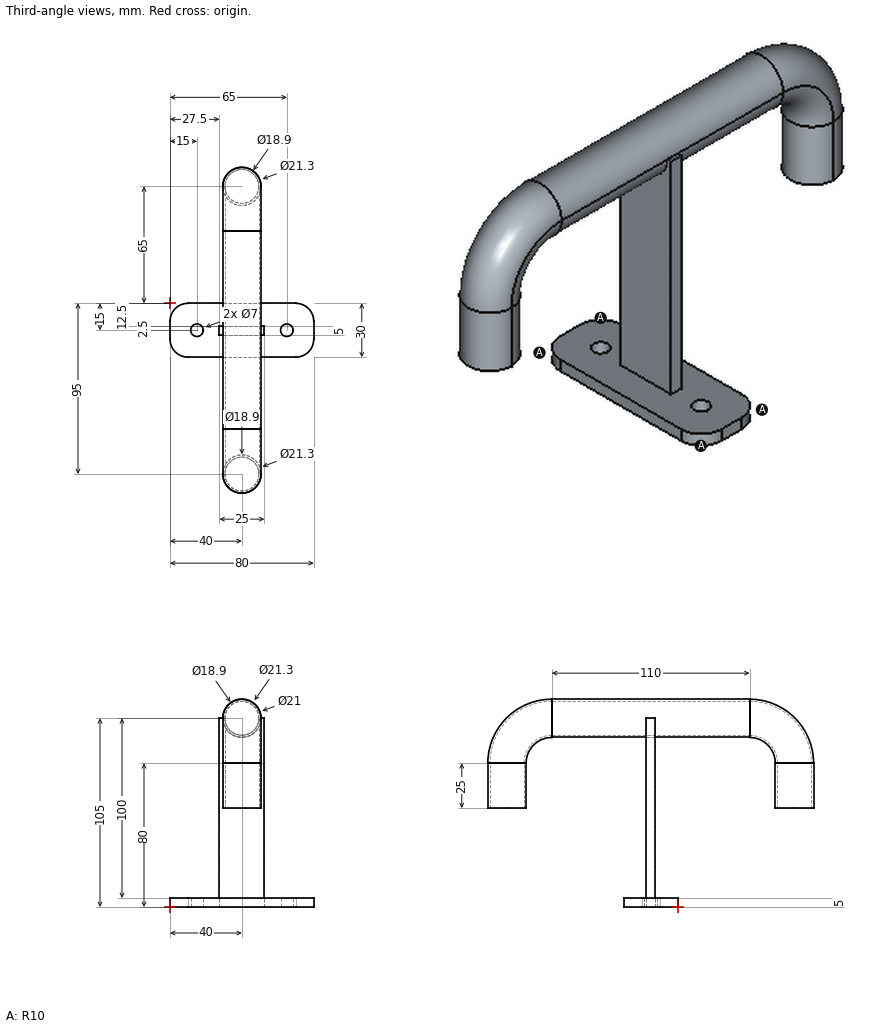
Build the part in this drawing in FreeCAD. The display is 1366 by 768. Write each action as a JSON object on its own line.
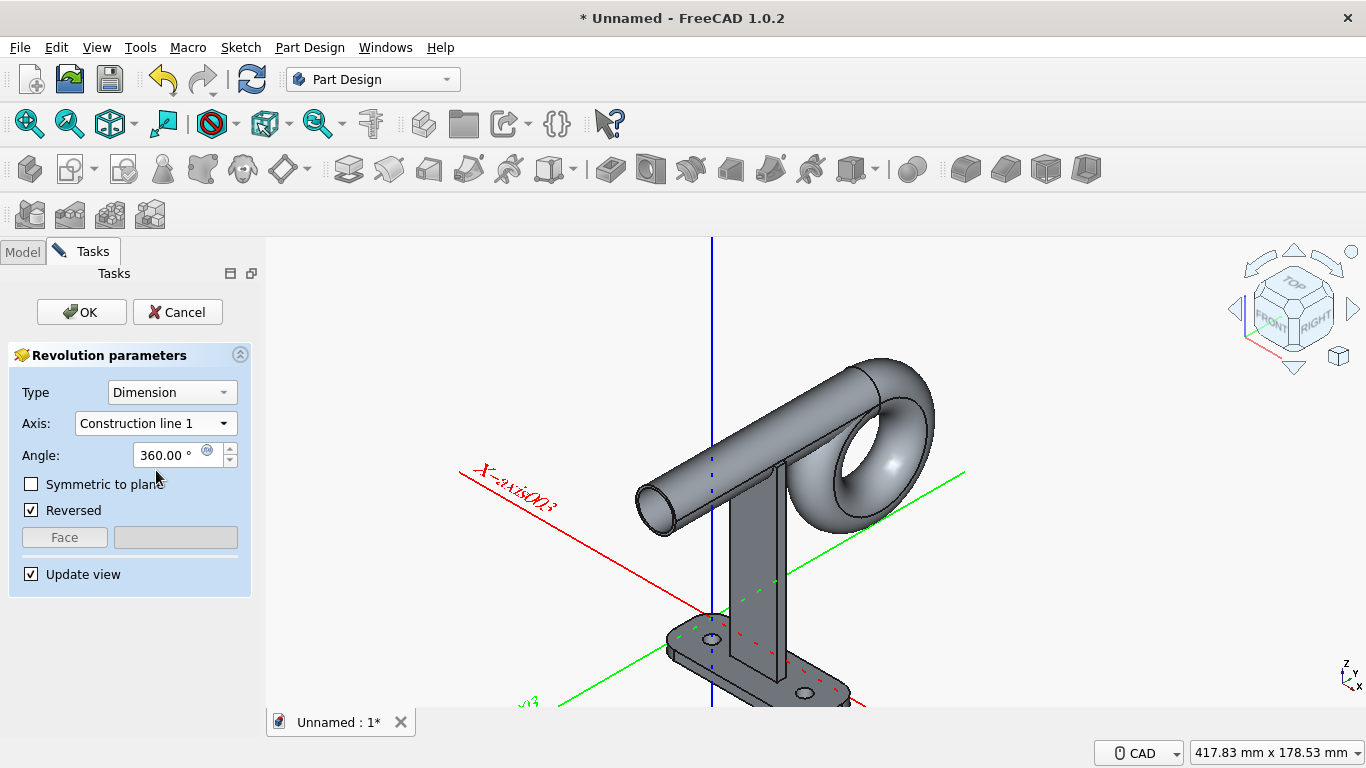
{"action": "triple_click", "coordinate": [178, 455]}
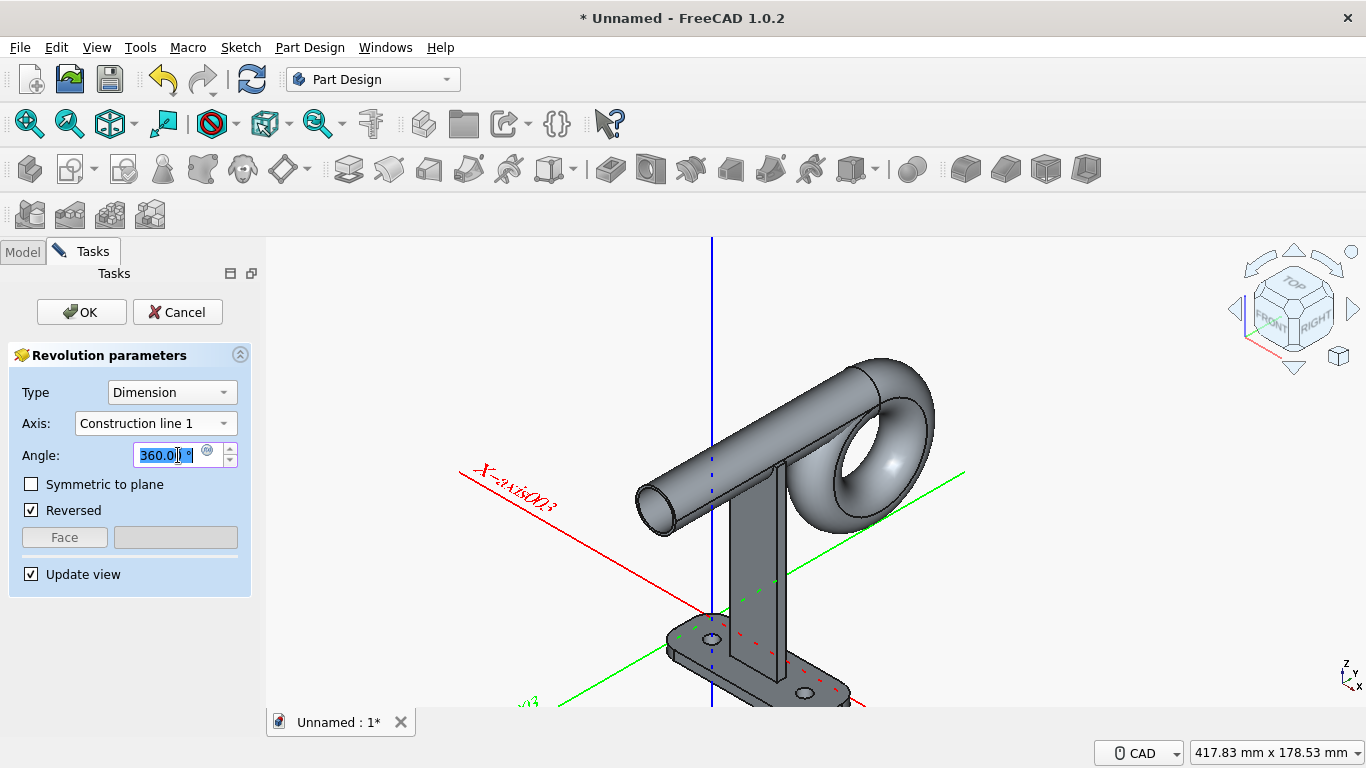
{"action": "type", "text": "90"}
{"action": "key", "text": "Tab"}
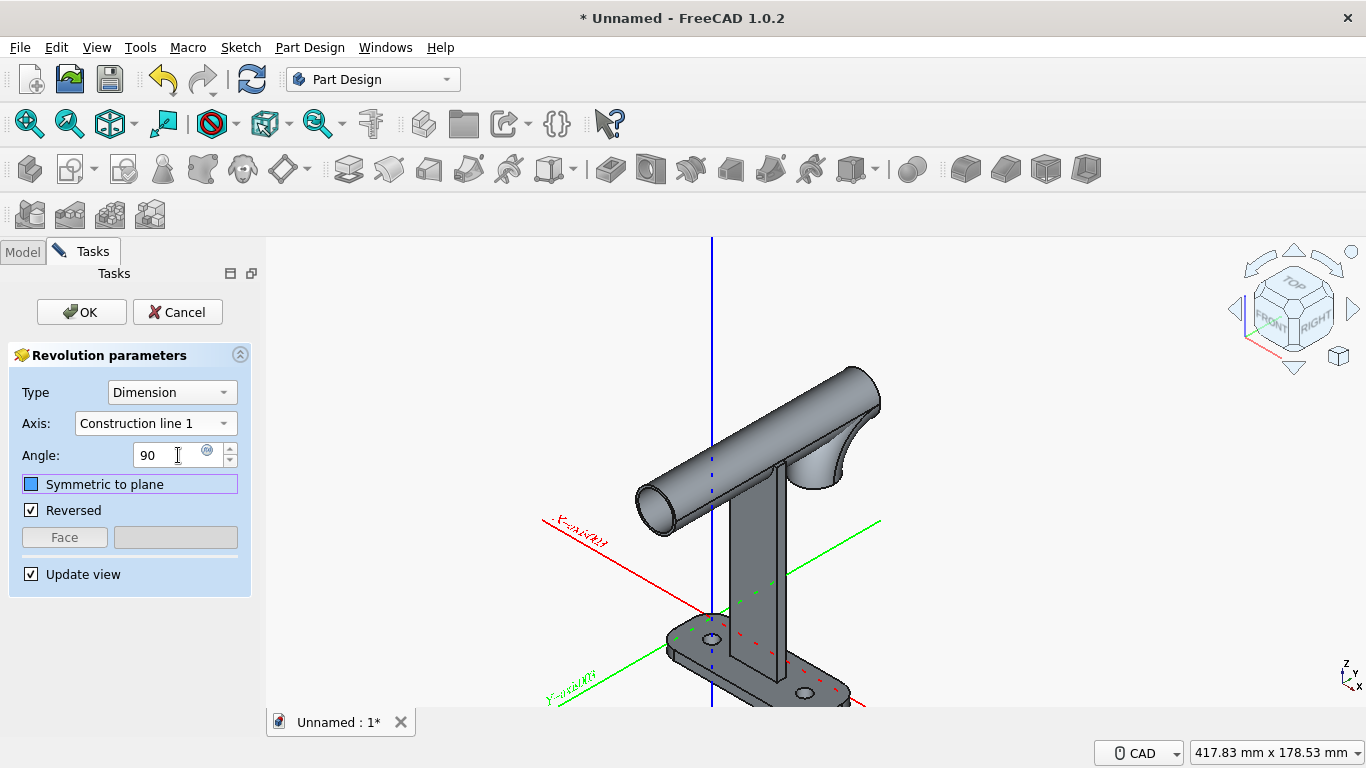
{"action": "left_click", "coordinate": [30, 510]}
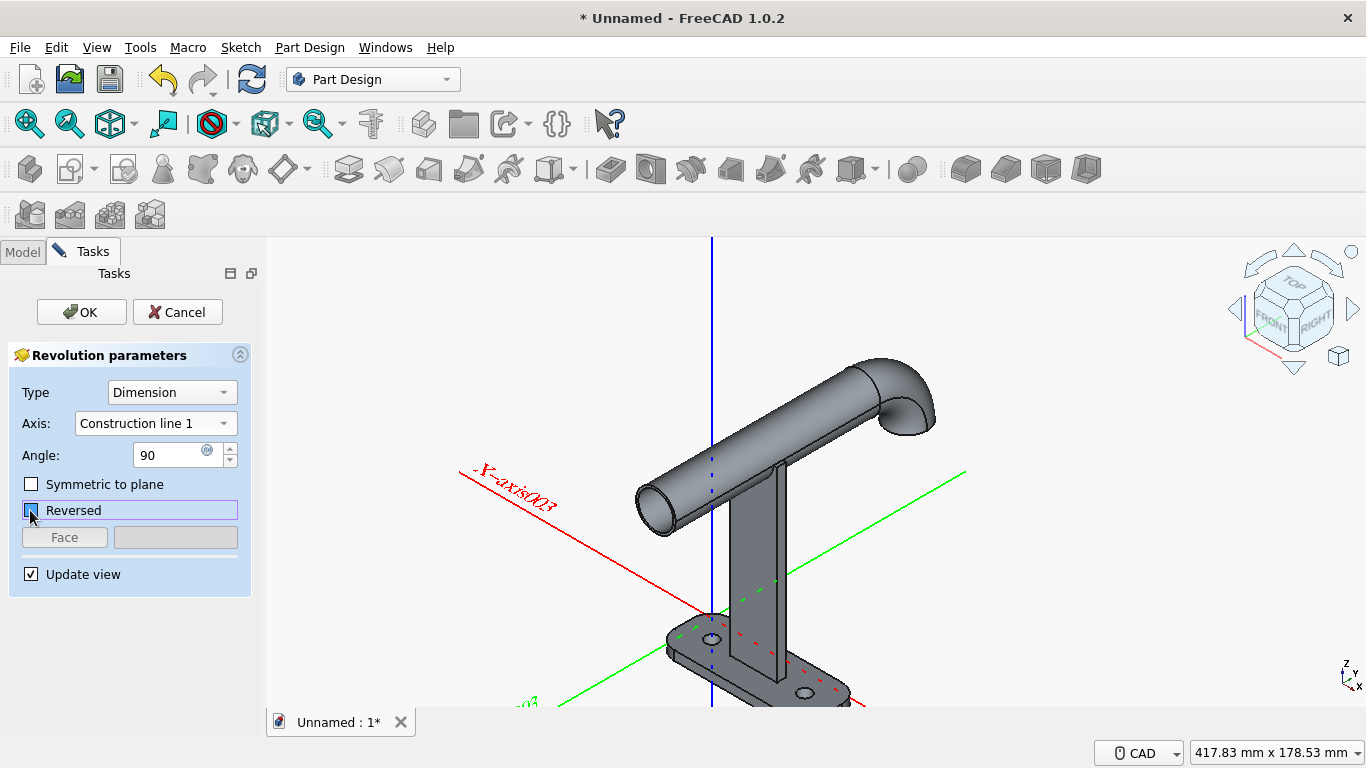
{"action": "left_click", "coordinate": [82, 312]}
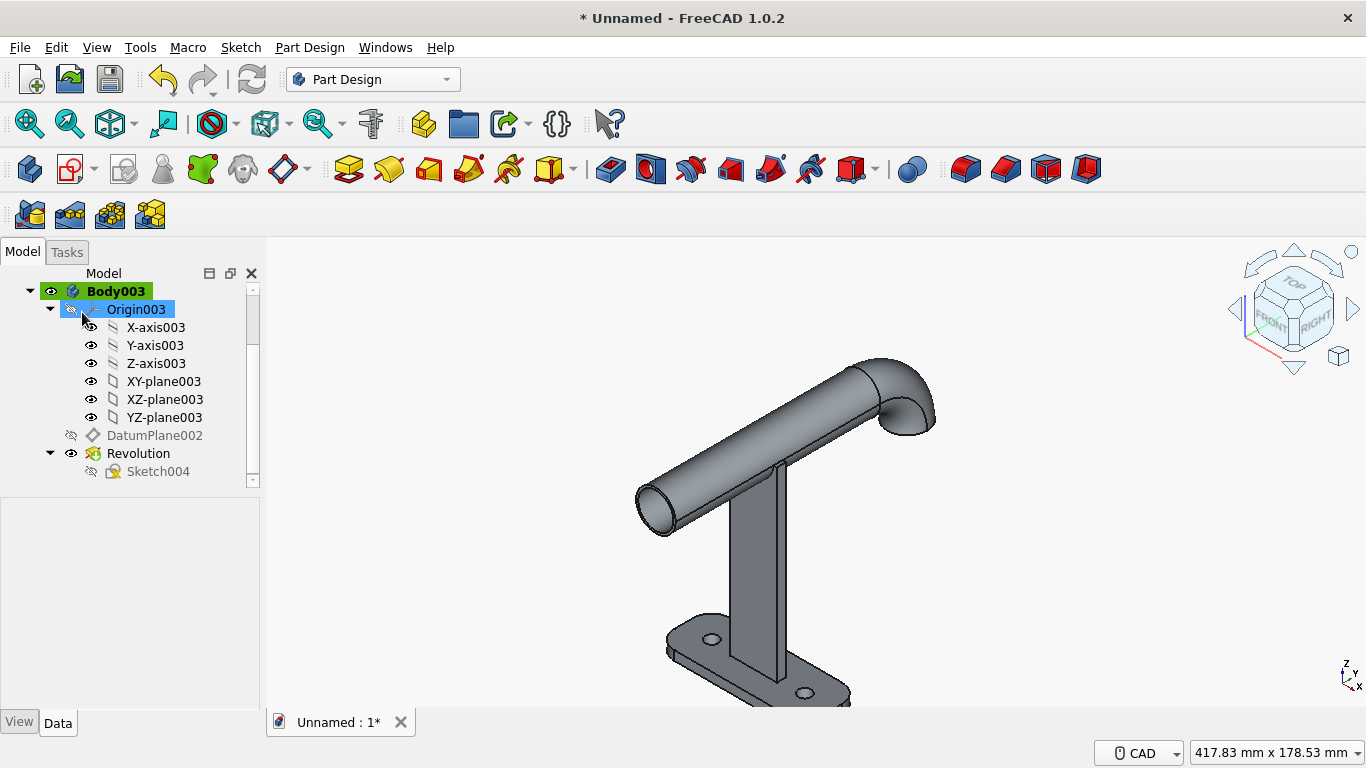
{"action": "left_click", "coordinate": [30, 124]}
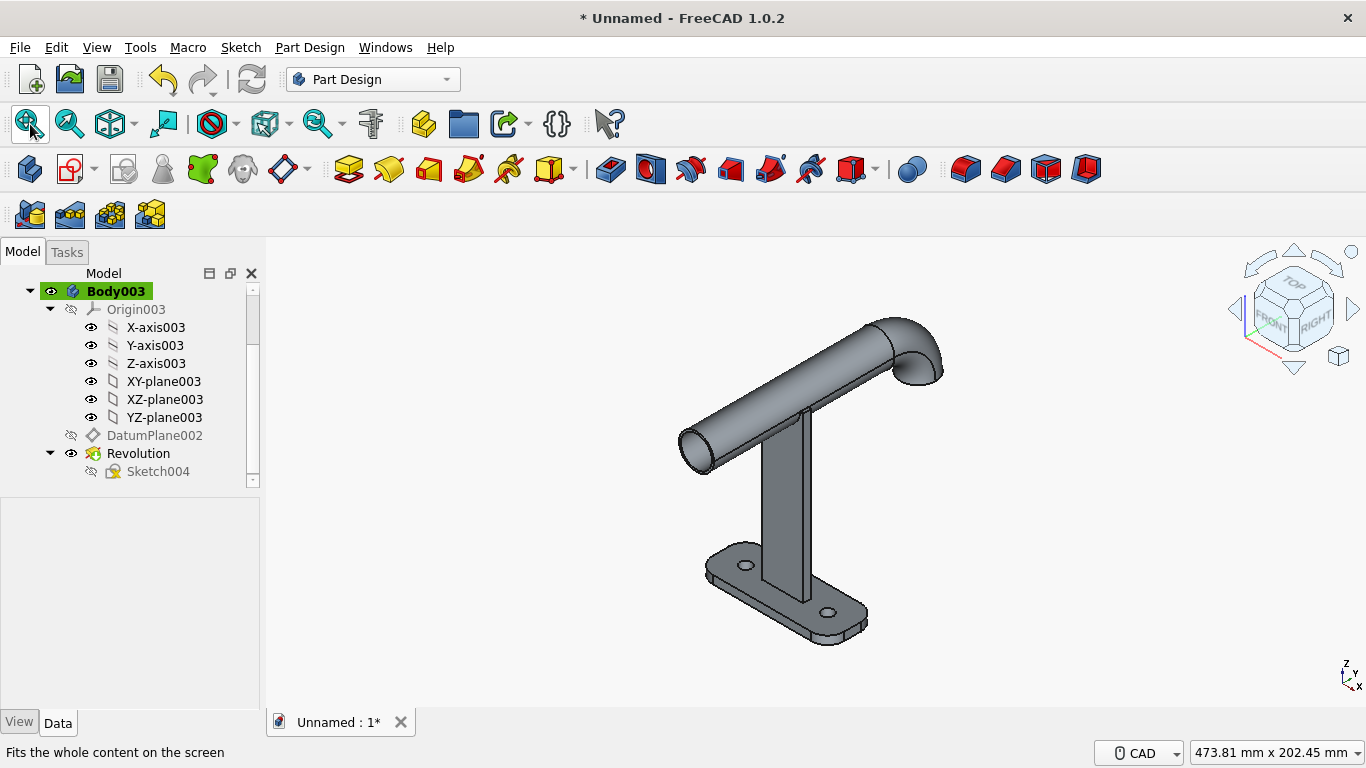
{"action": "left_click", "coordinate": [30, 170]}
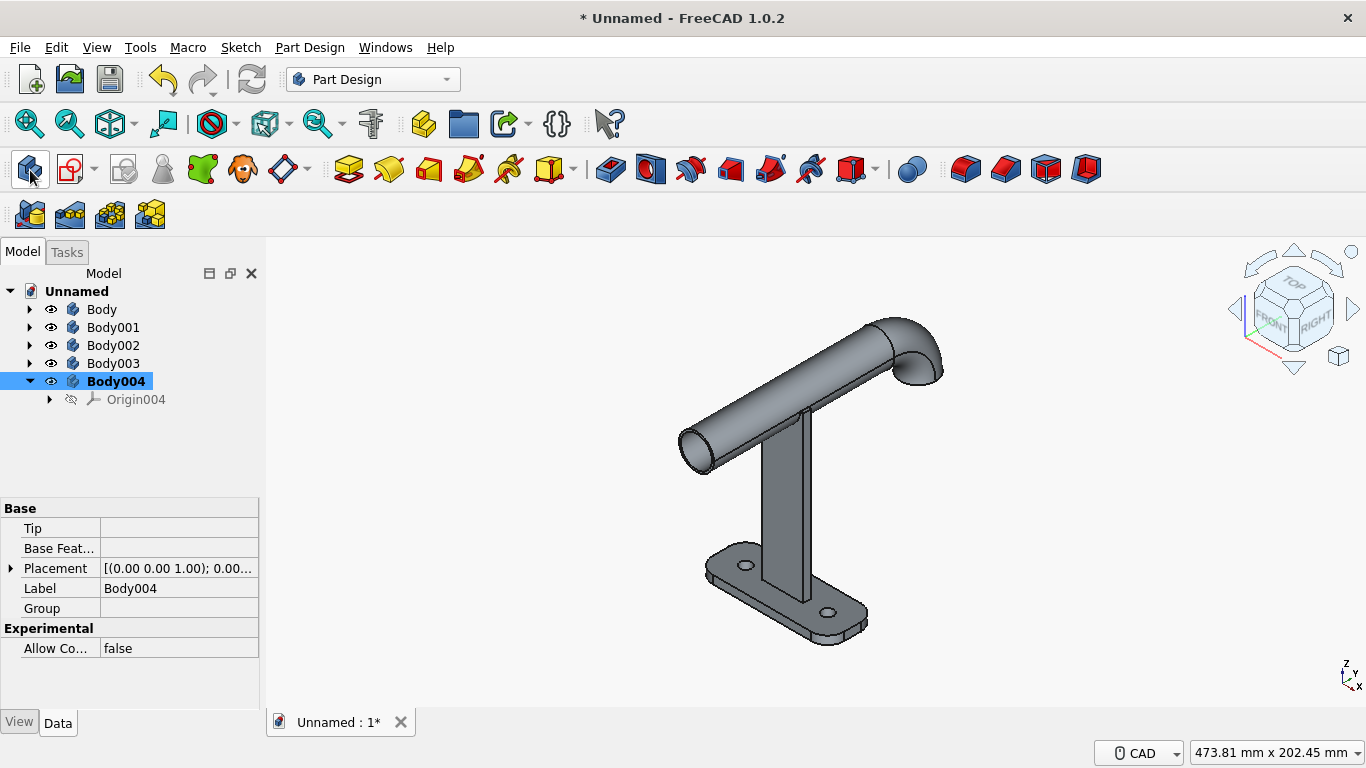
{"action": "left_click", "coordinate": [50, 399]}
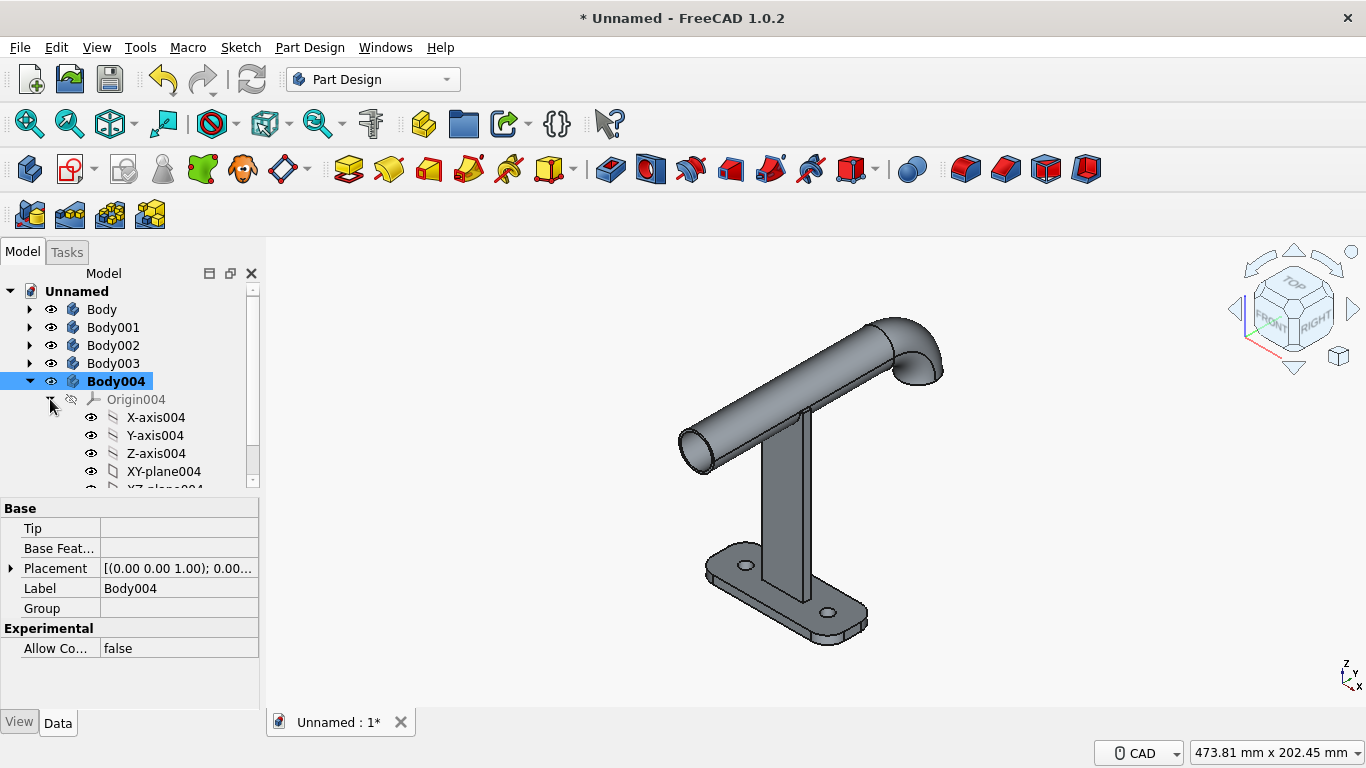
{"action": "scroll", "coordinate": [100, 377], "scroll_direction": "down", "scroll_amount": 3}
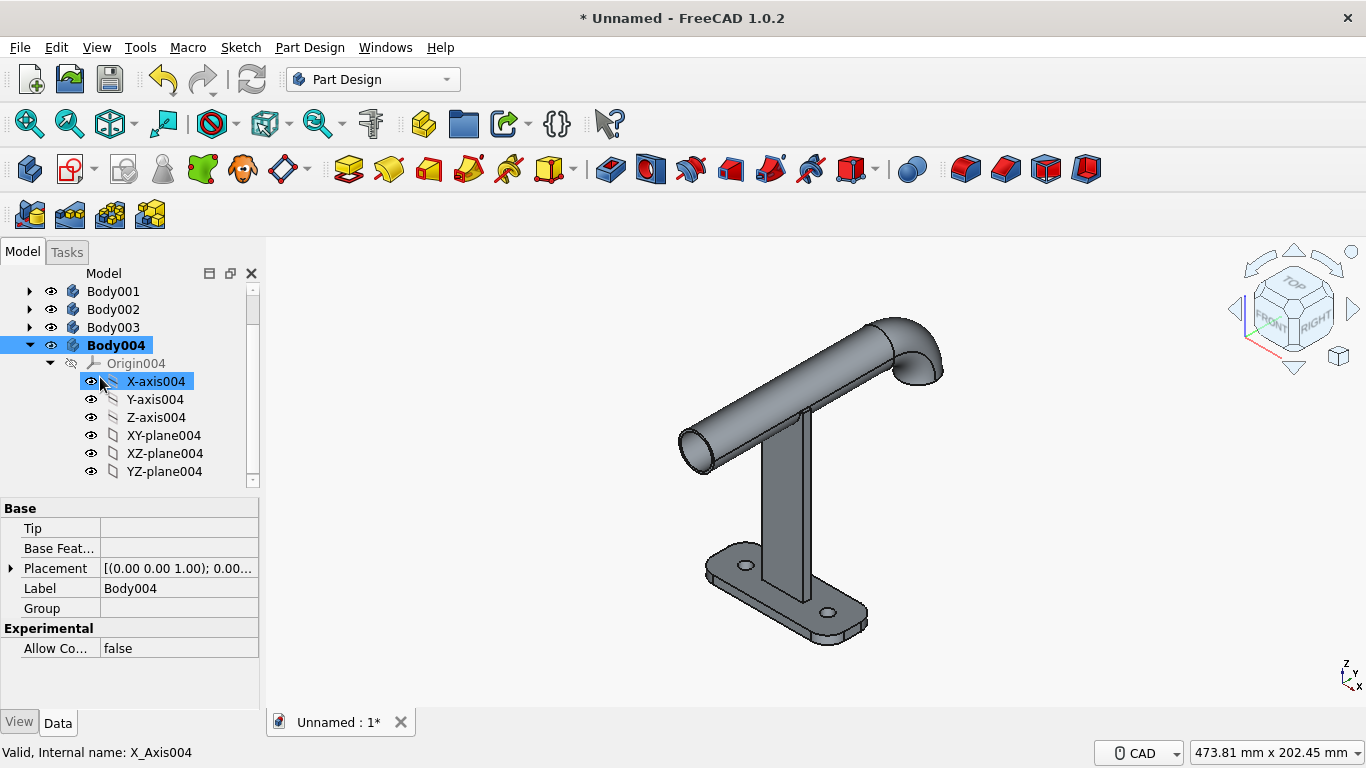
{"action": "left_click", "coordinate": [136, 453]}